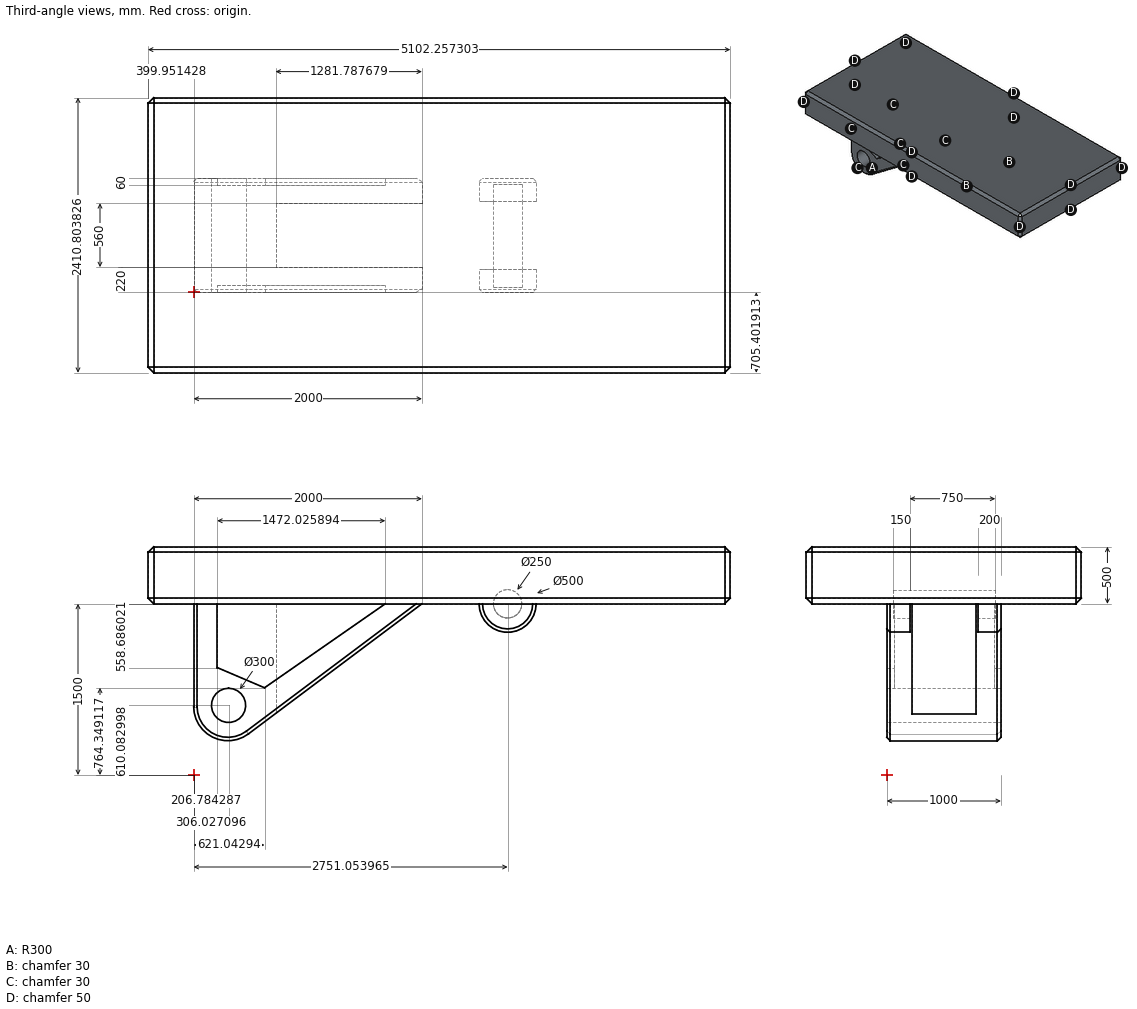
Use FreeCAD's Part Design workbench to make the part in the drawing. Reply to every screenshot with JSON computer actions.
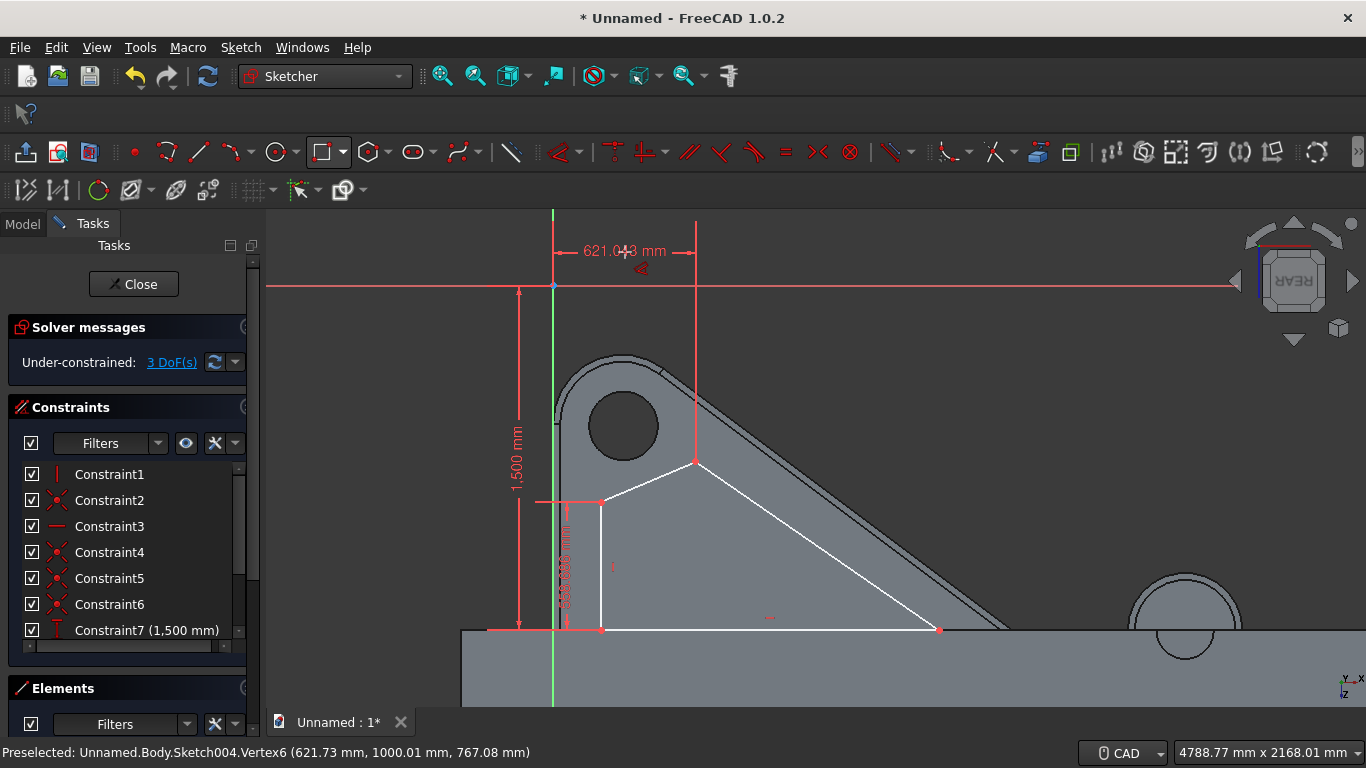
{"action": "left_click", "coordinate": [702, 630]}
{"action": "left_click", "coordinate": [770, 664]}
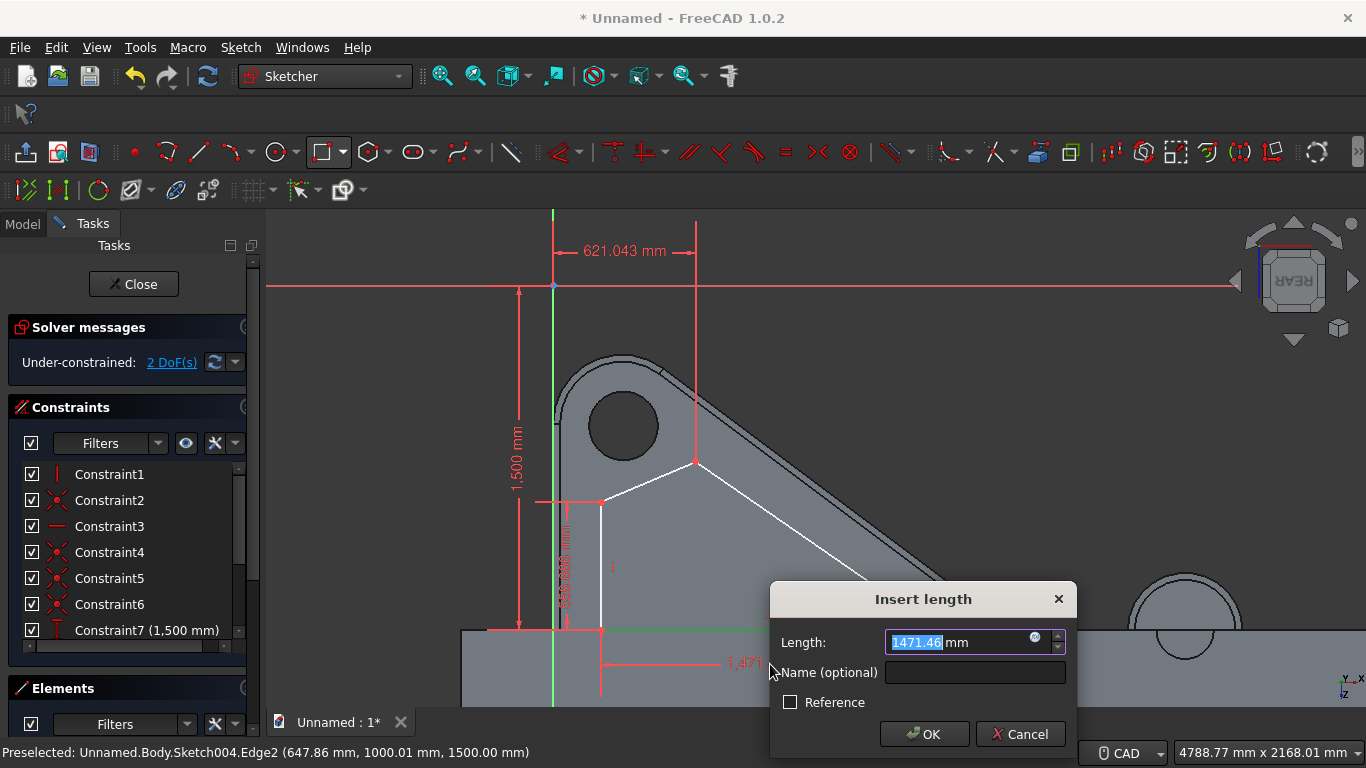
{"action": "type", "text": "1472.025894"}
{"action": "key", "text": "Return"}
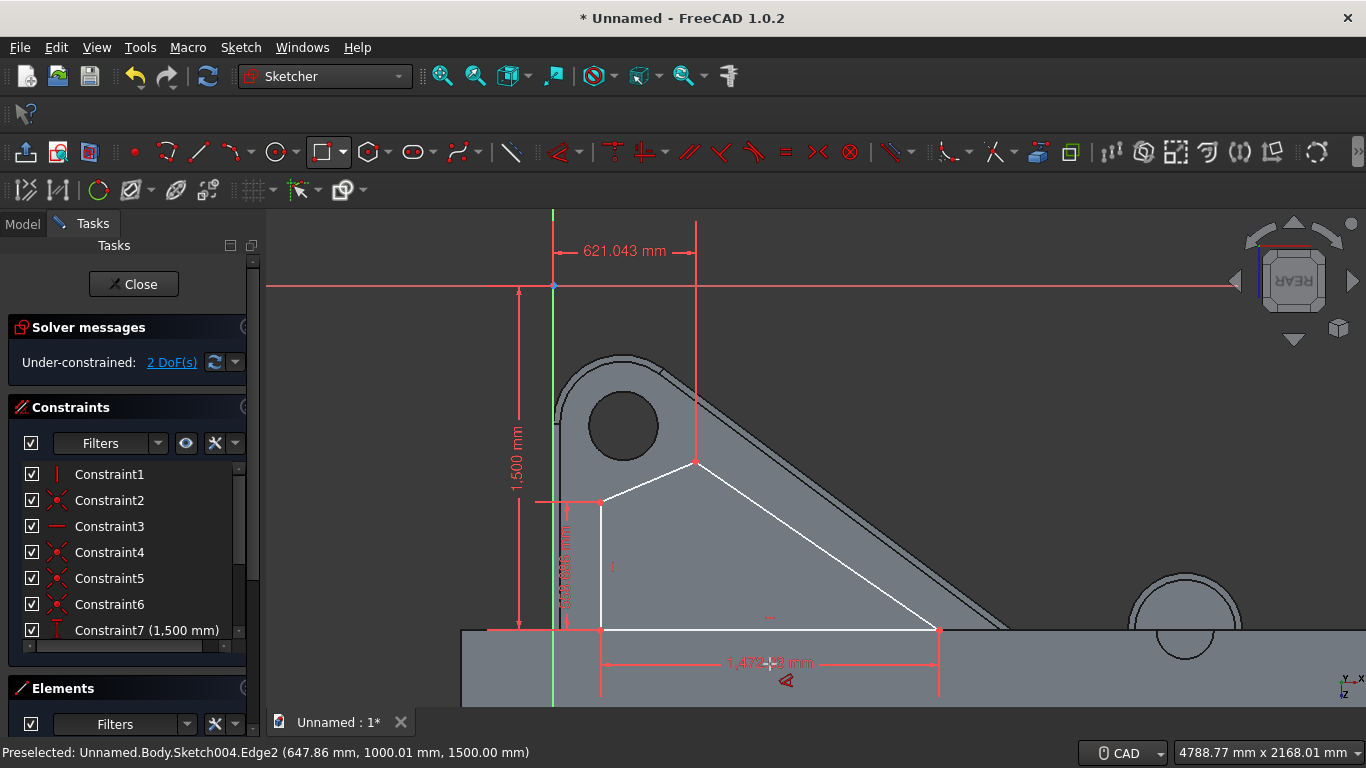
{"action": "left_click", "coordinate": [601, 502]}
{"action": "left_click", "coordinate": [577, 536]}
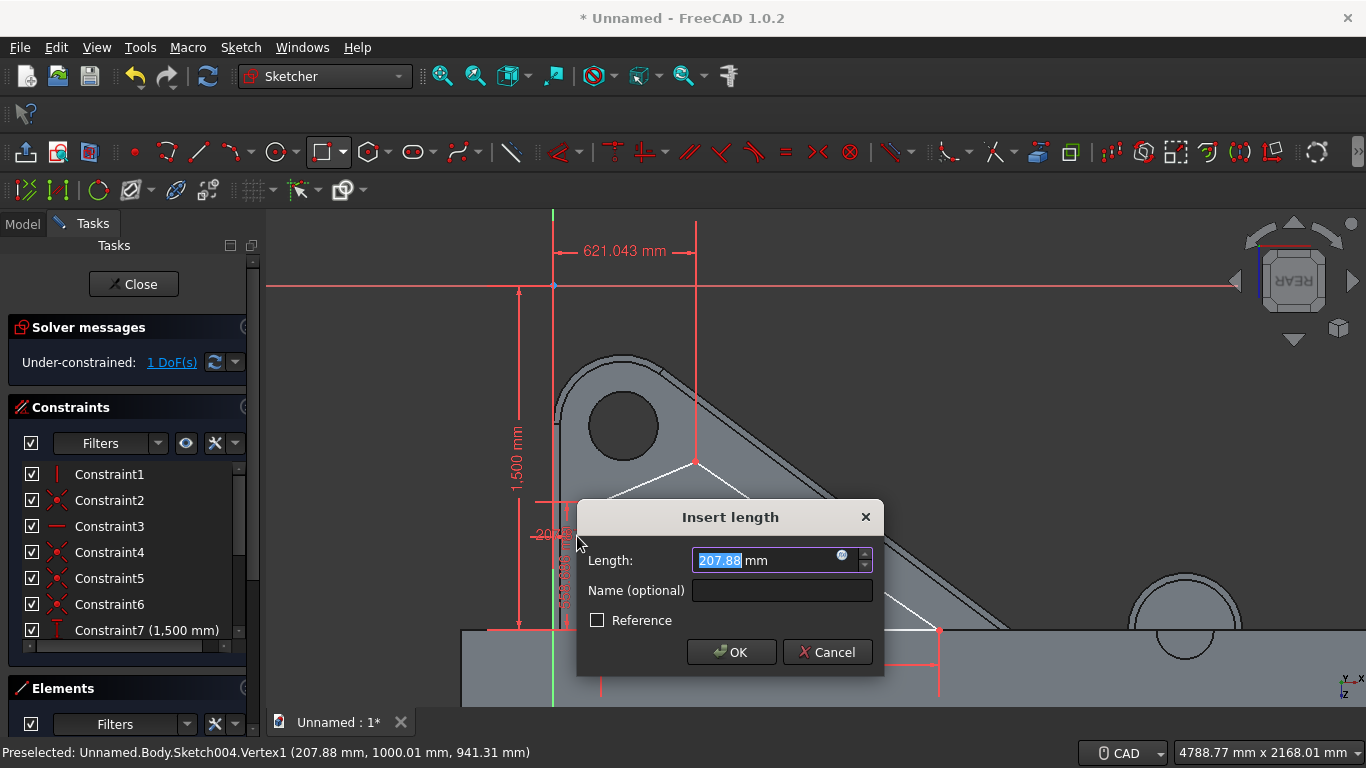
{"action": "type", "text": "206.784287"}
{"action": "key", "text": "Return"}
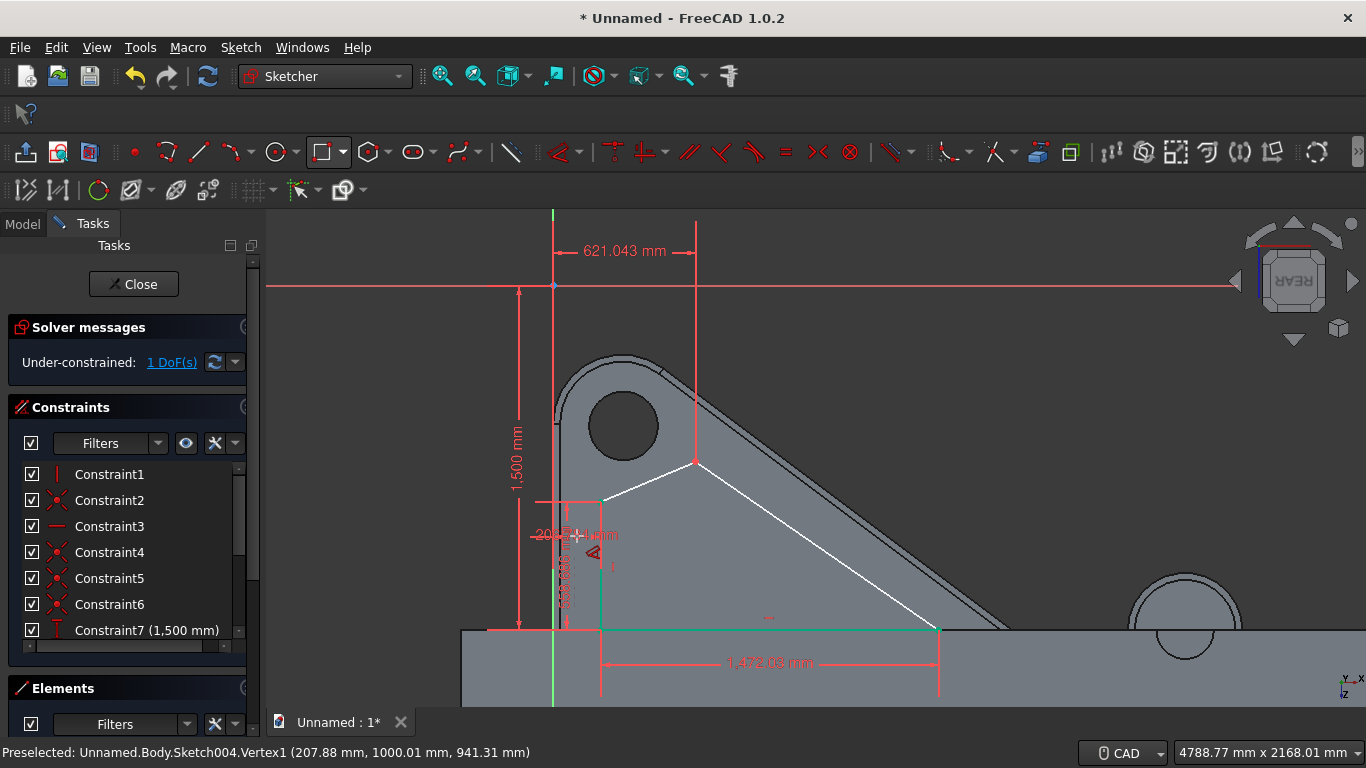
{"action": "left_click", "coordinate": [696, 462]}
{"action": "left_click", "coordinate": [519, 374]}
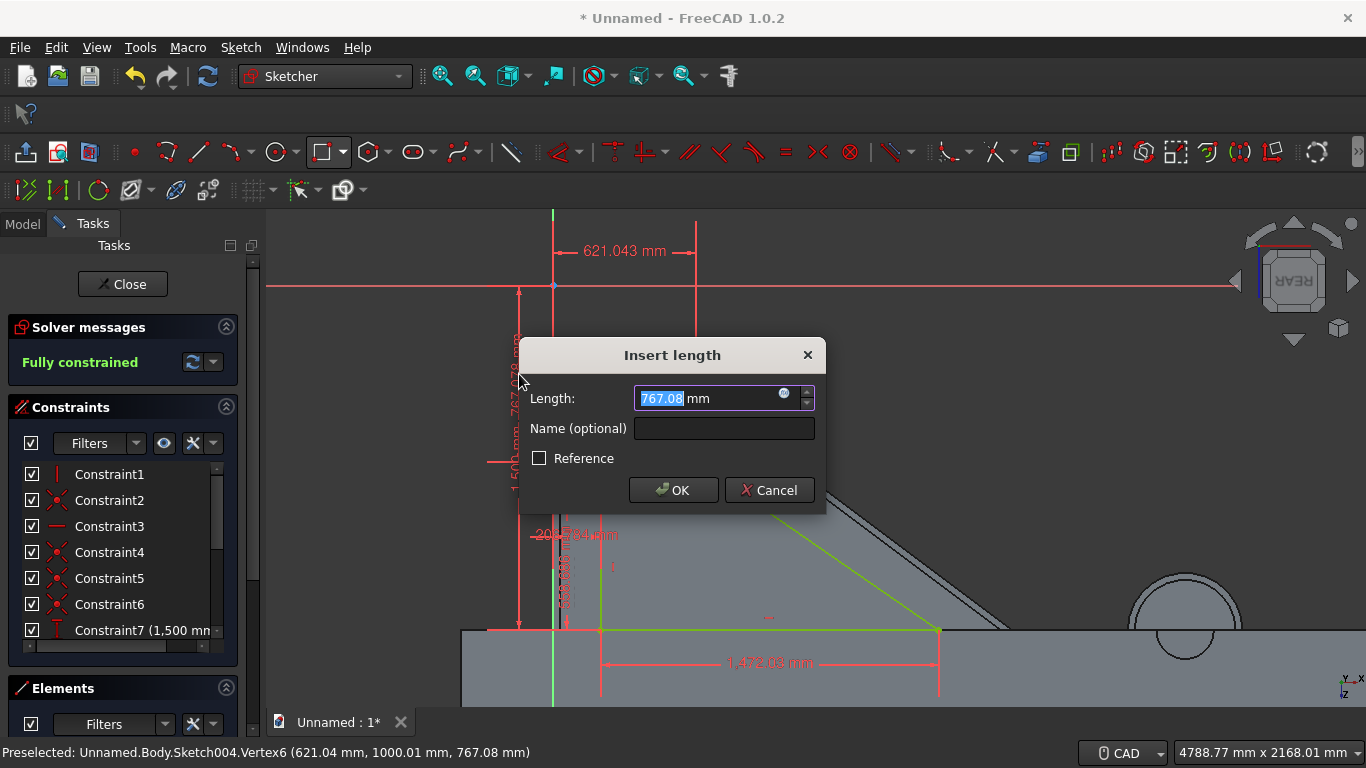
{"action": "type", "text": "764.349117"}
{"action": "key", "text": "Return"}
{"action": "key", "text": "Escape"}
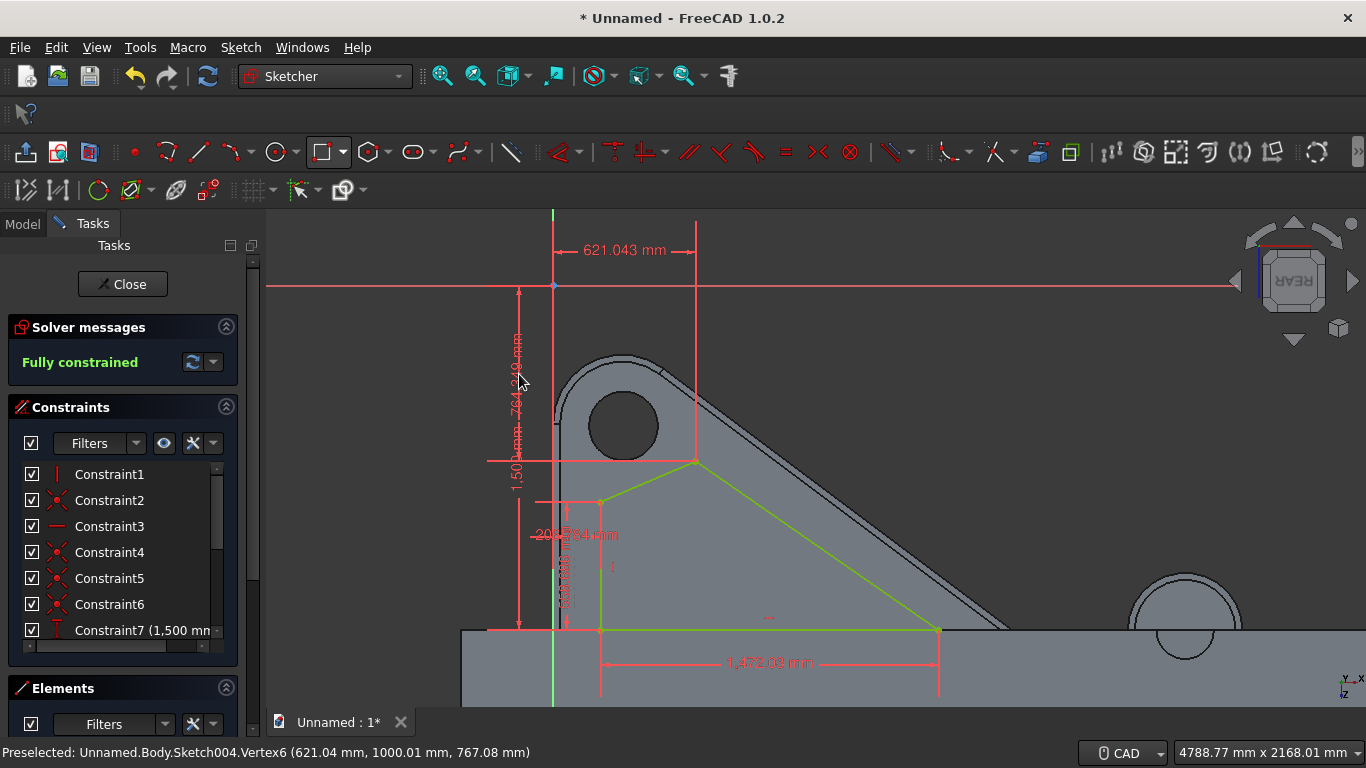
{"action": "left_click", "coordinate": [123, 284]}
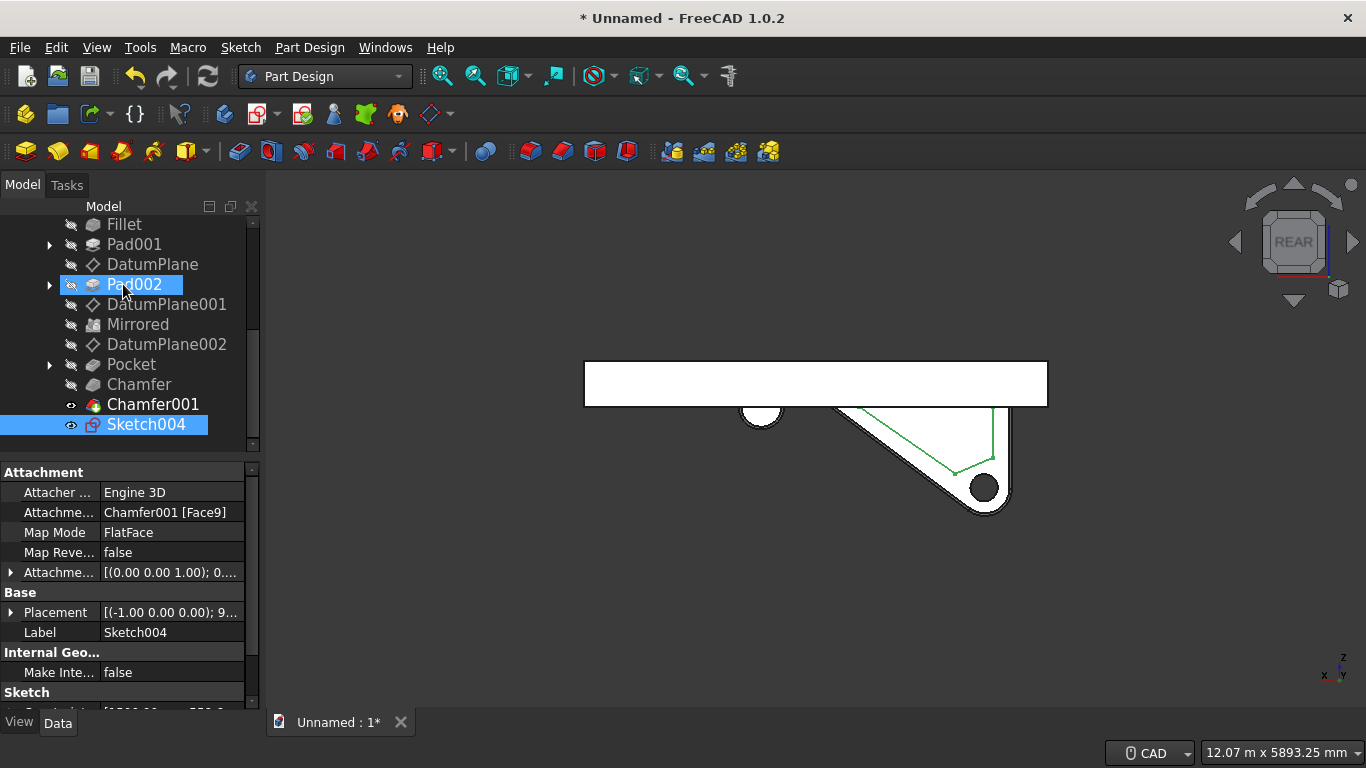
{"action": "left_click", "coordinate": [240, 152]}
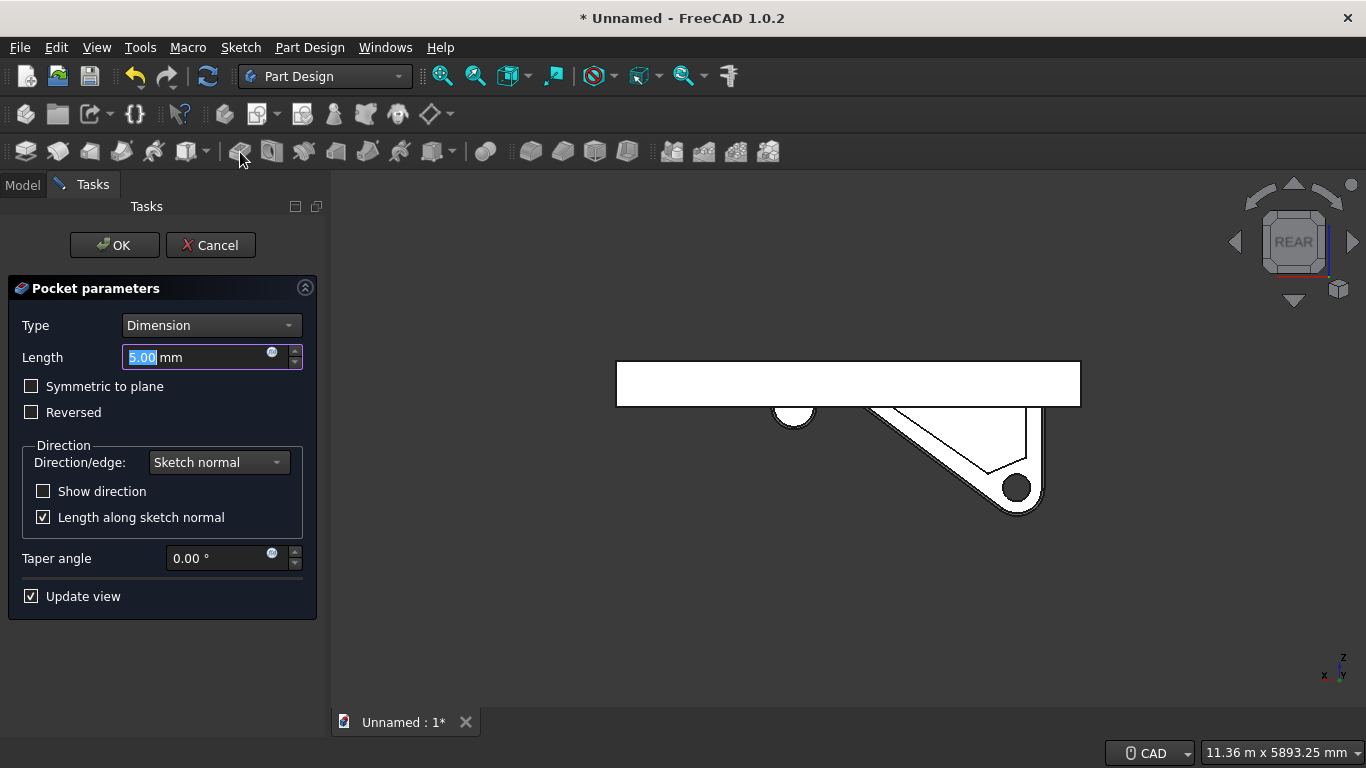
{"action": "type", "text": "60"}
{"action": "key", "text": "Tab"}